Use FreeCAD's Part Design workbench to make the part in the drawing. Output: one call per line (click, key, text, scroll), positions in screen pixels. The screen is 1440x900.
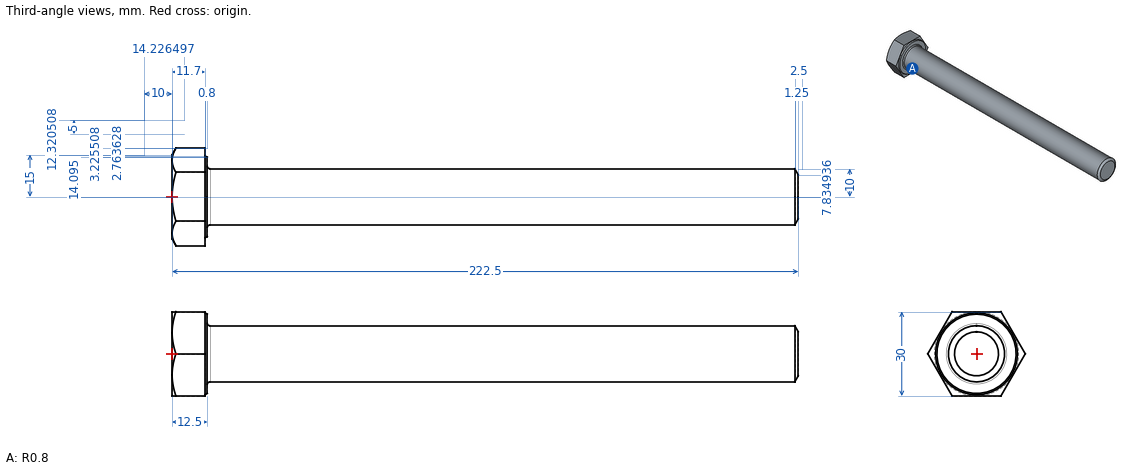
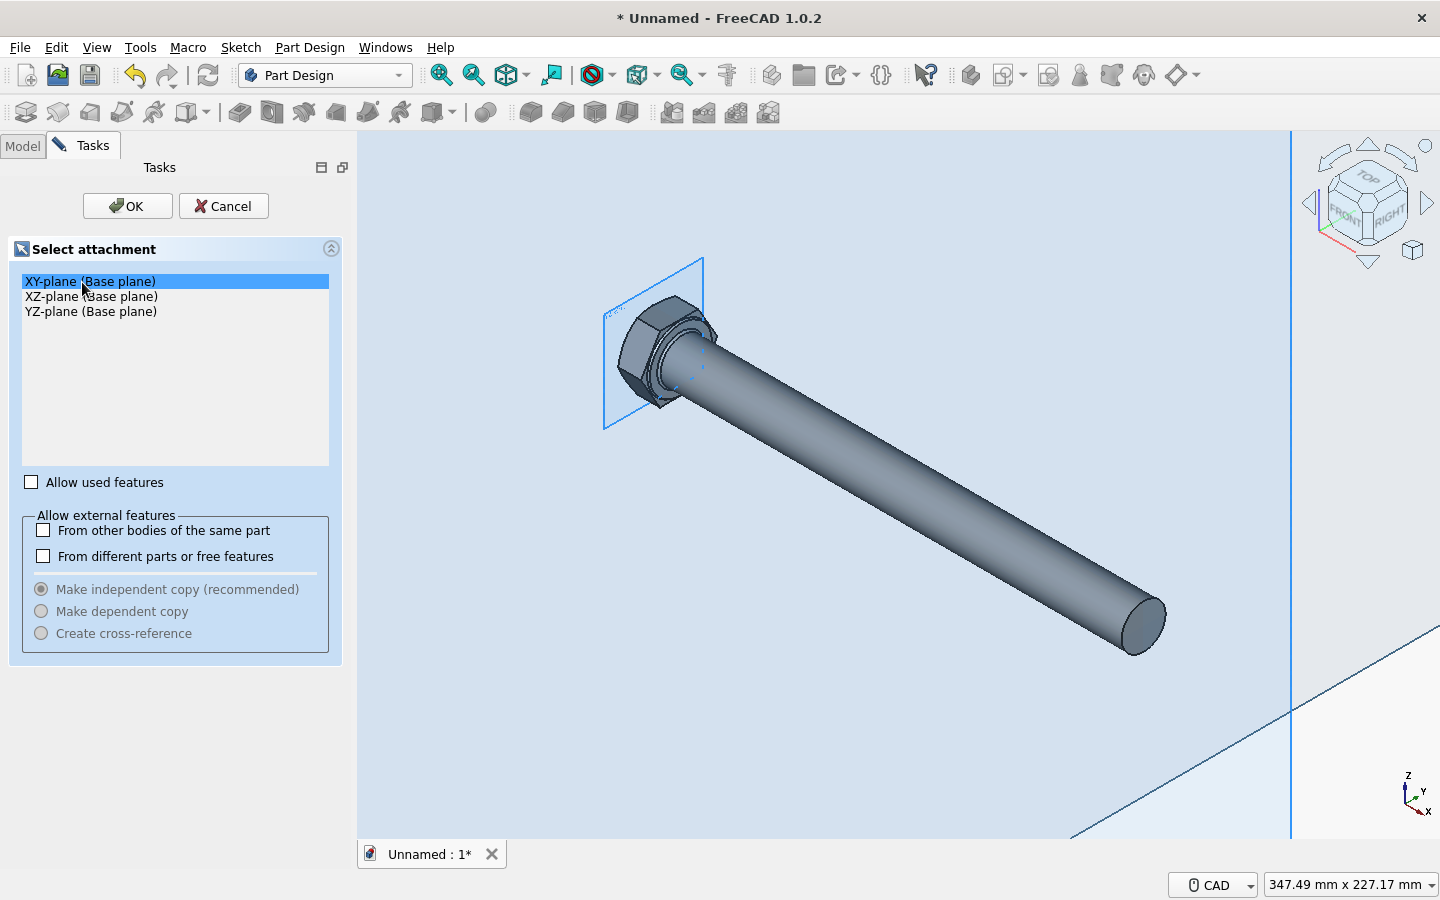
click(128, 206)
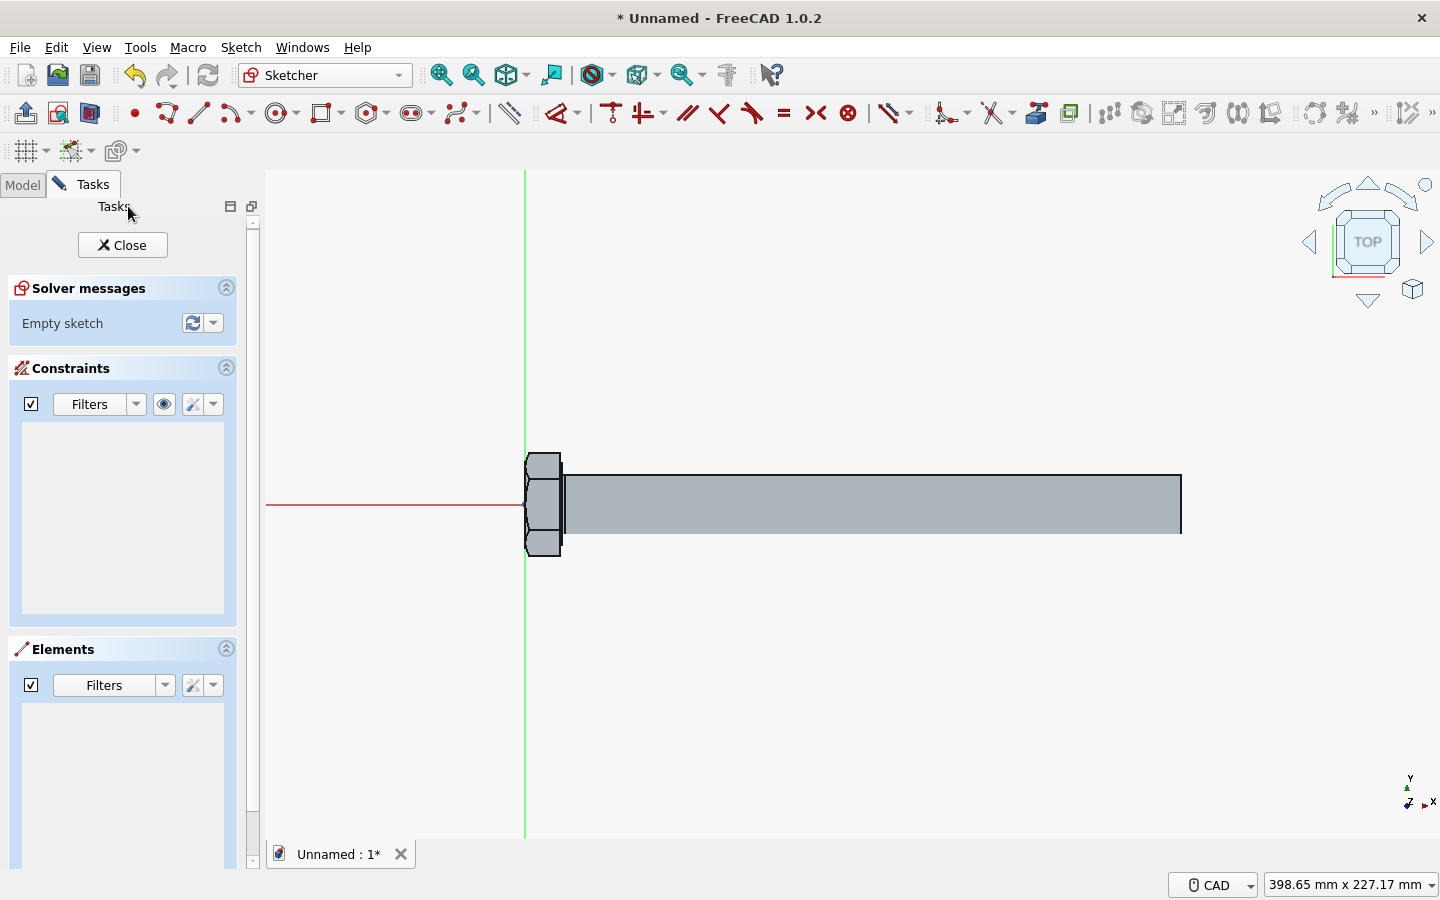
click(90, 114)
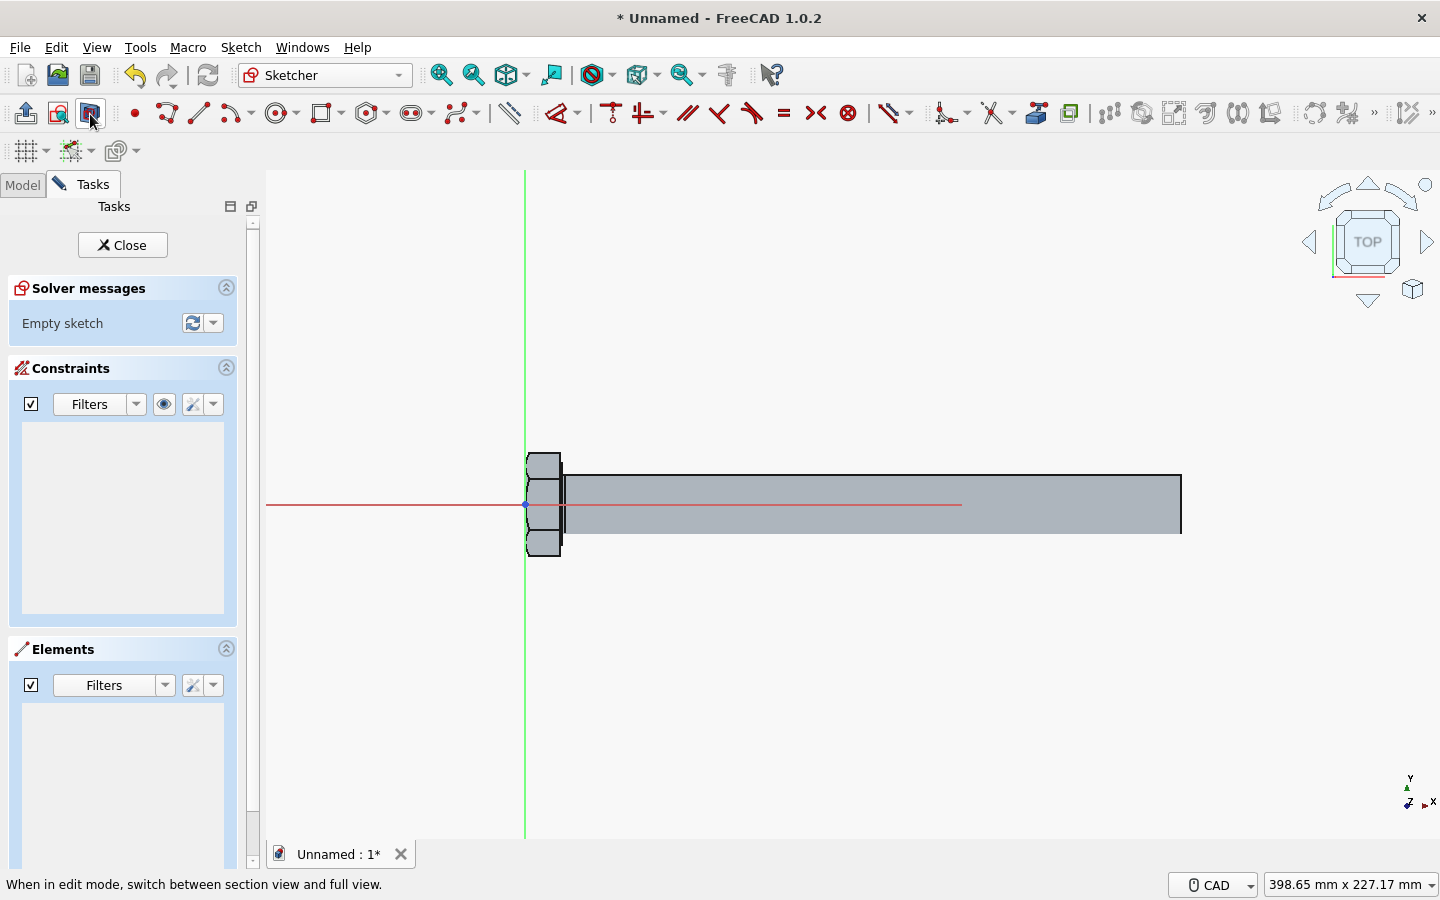
scroll(1201, 477, up, 15)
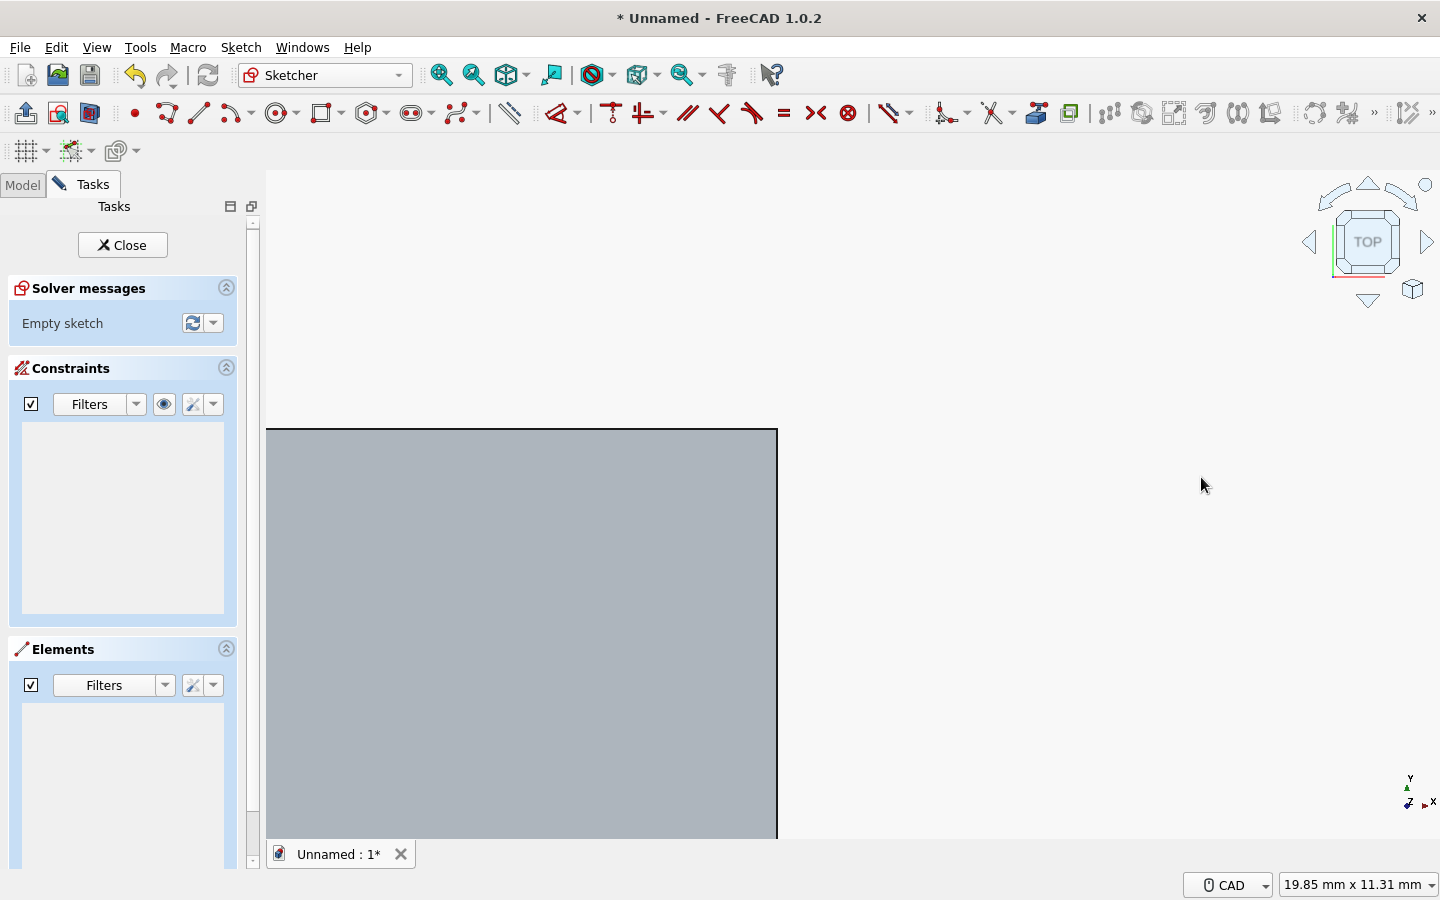
scroll(773, 488, up, 6)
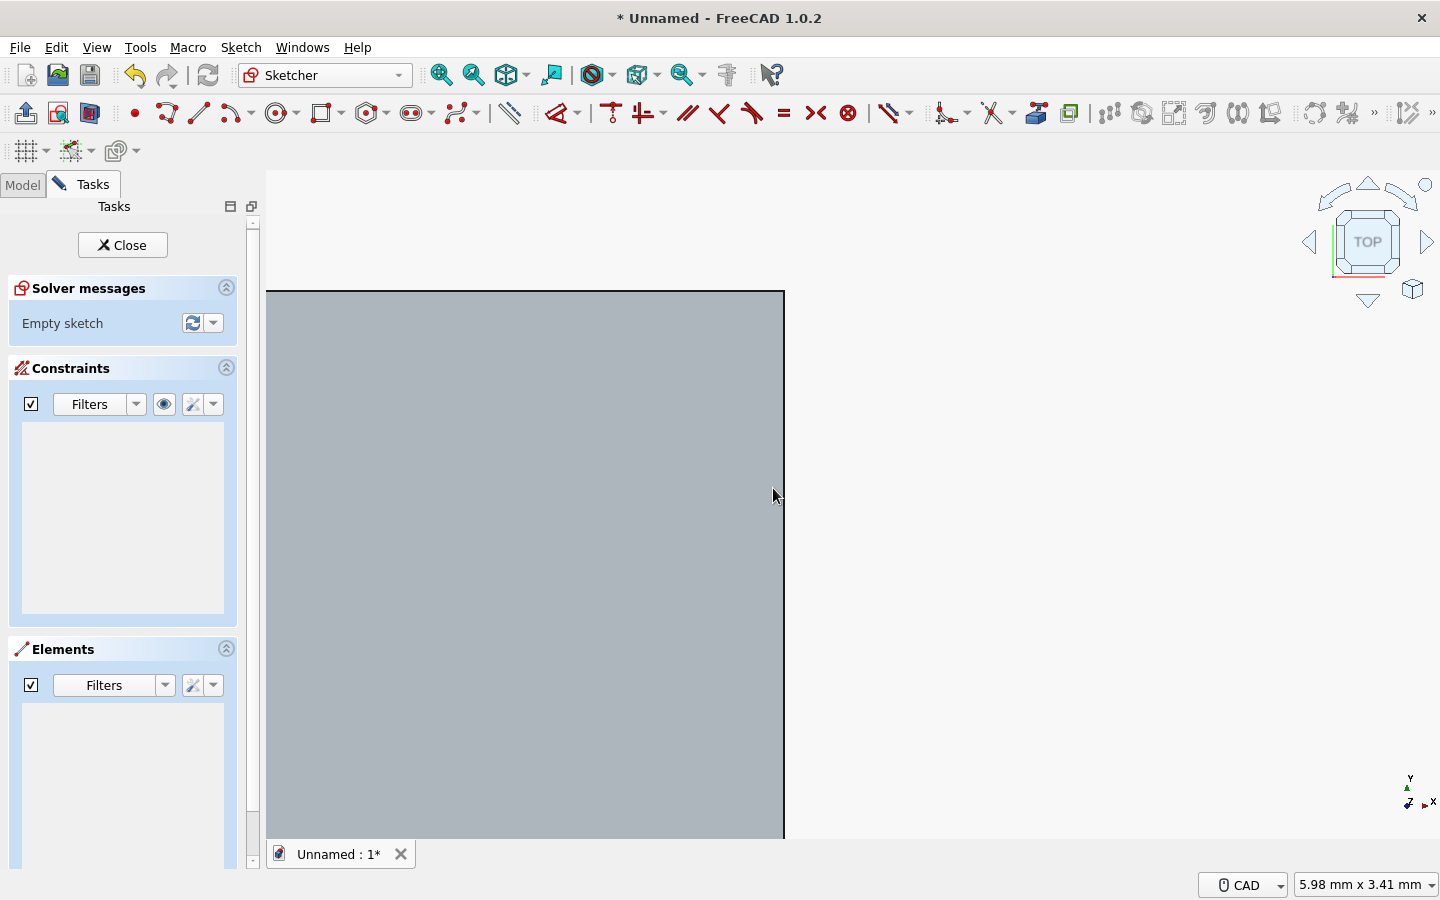
click(168, 114)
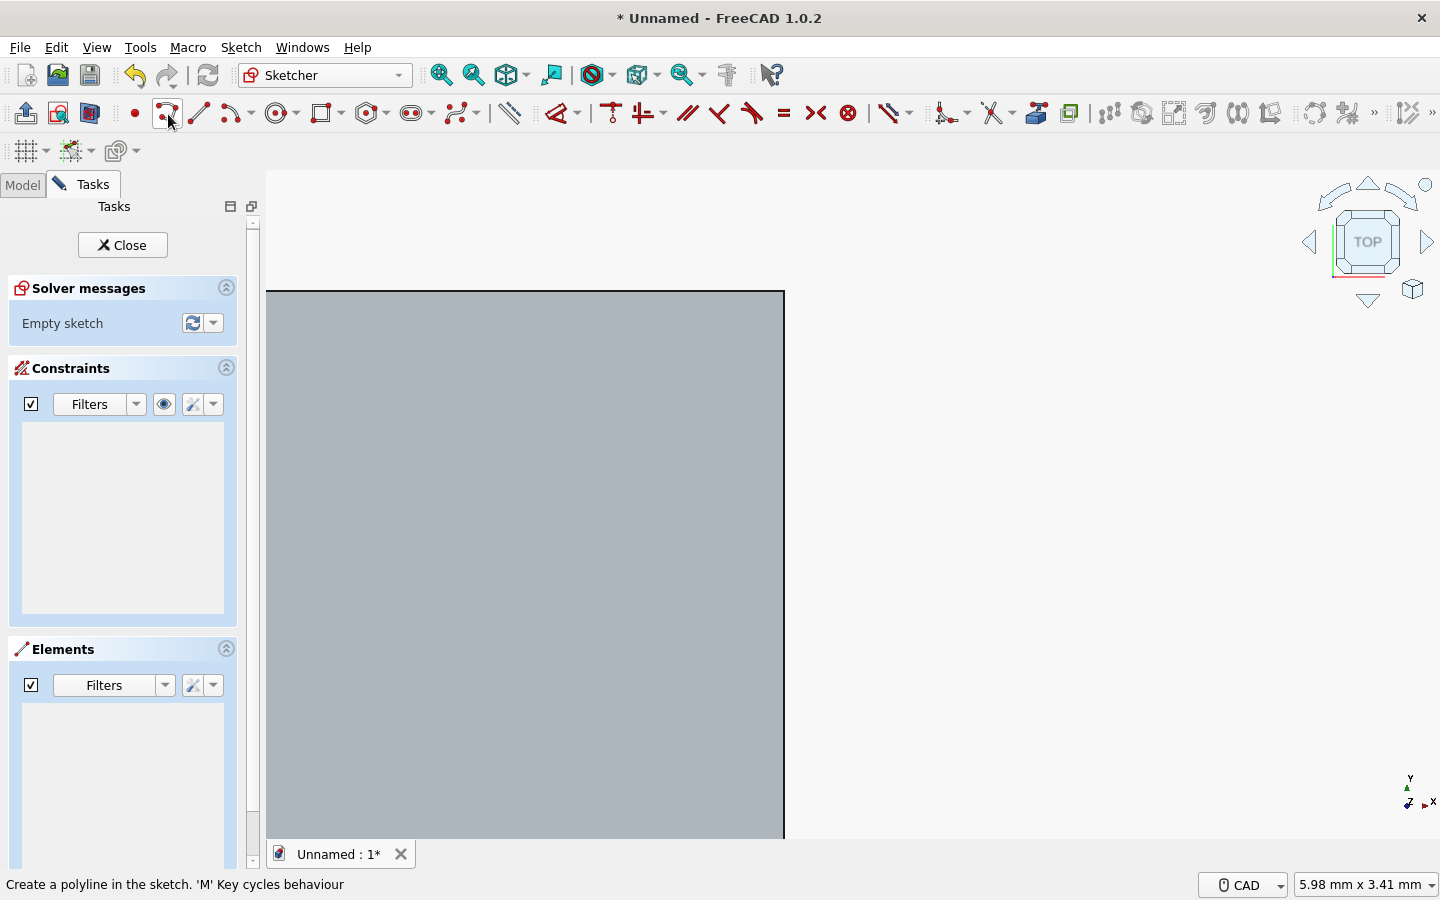
click(538, 291)
click(784, 716)
click(1029, 291)
click(538, 292)
key(Escape)
key(Escape)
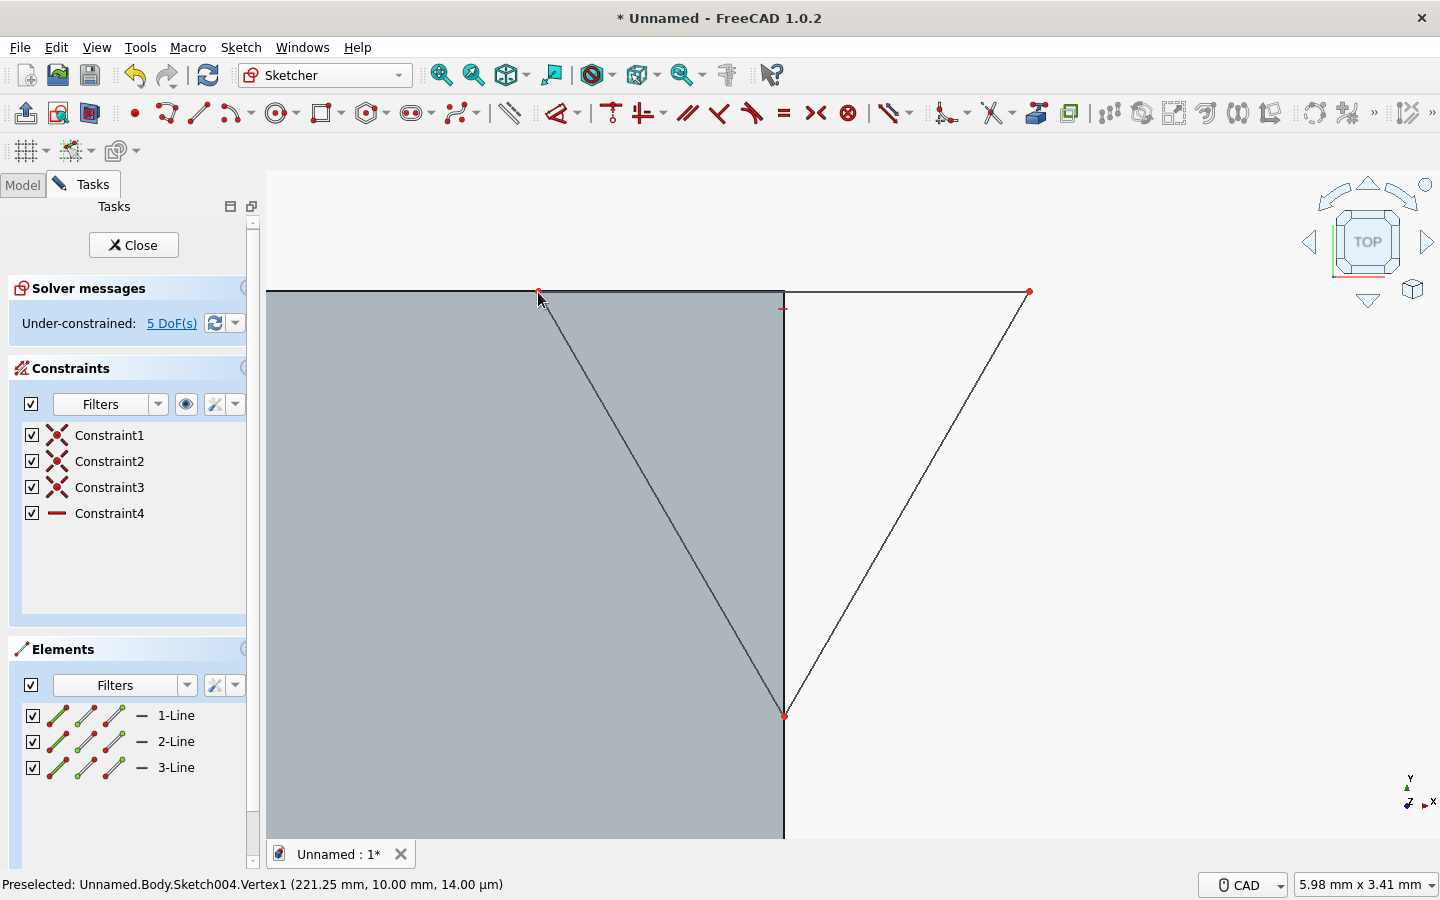
click(556, 114)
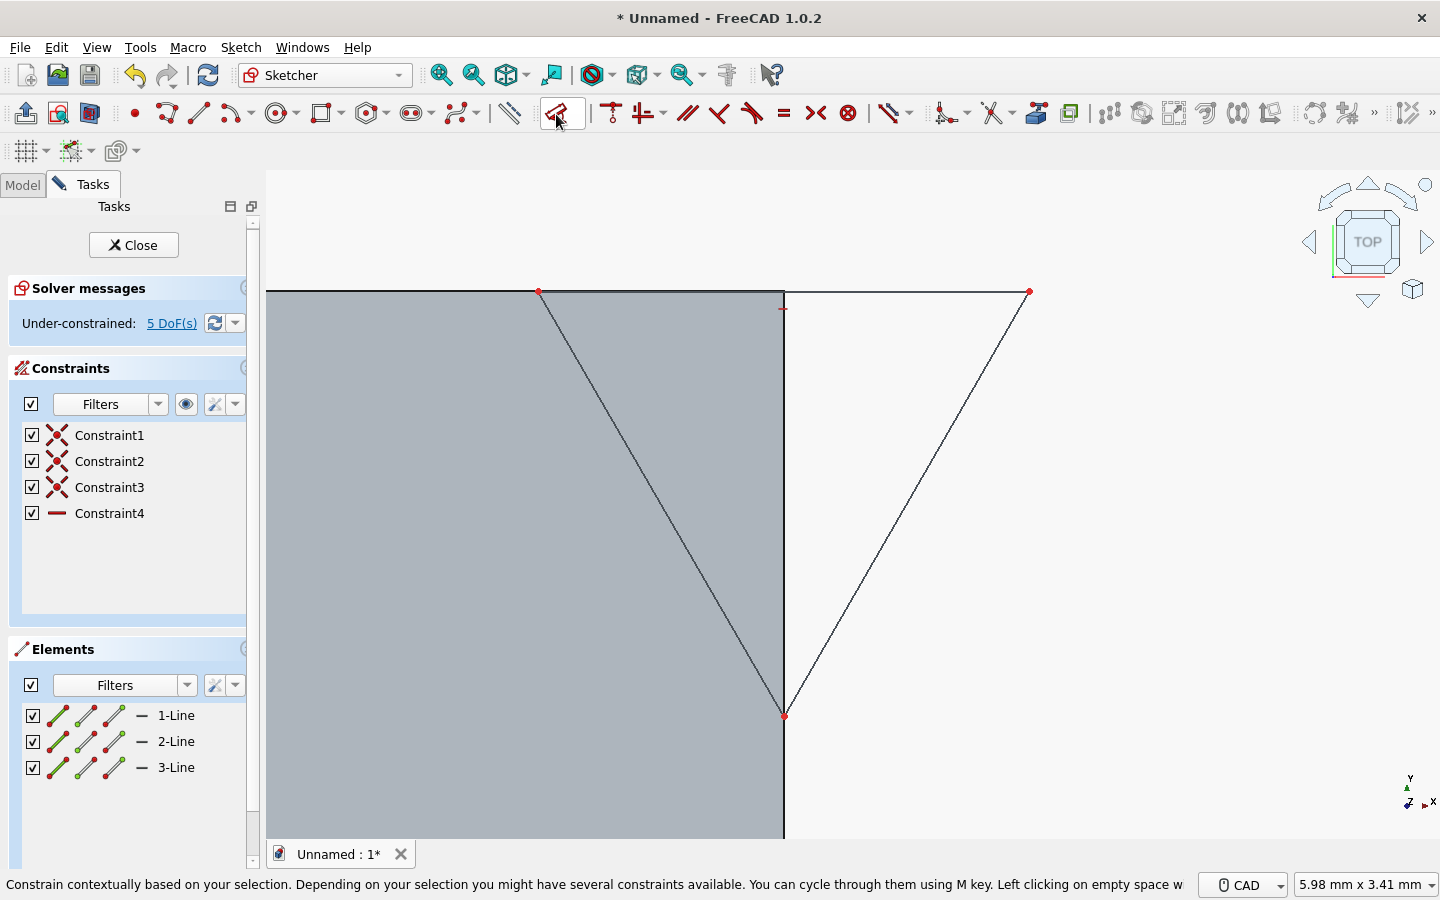
click(882, 292)
click(784, 258)